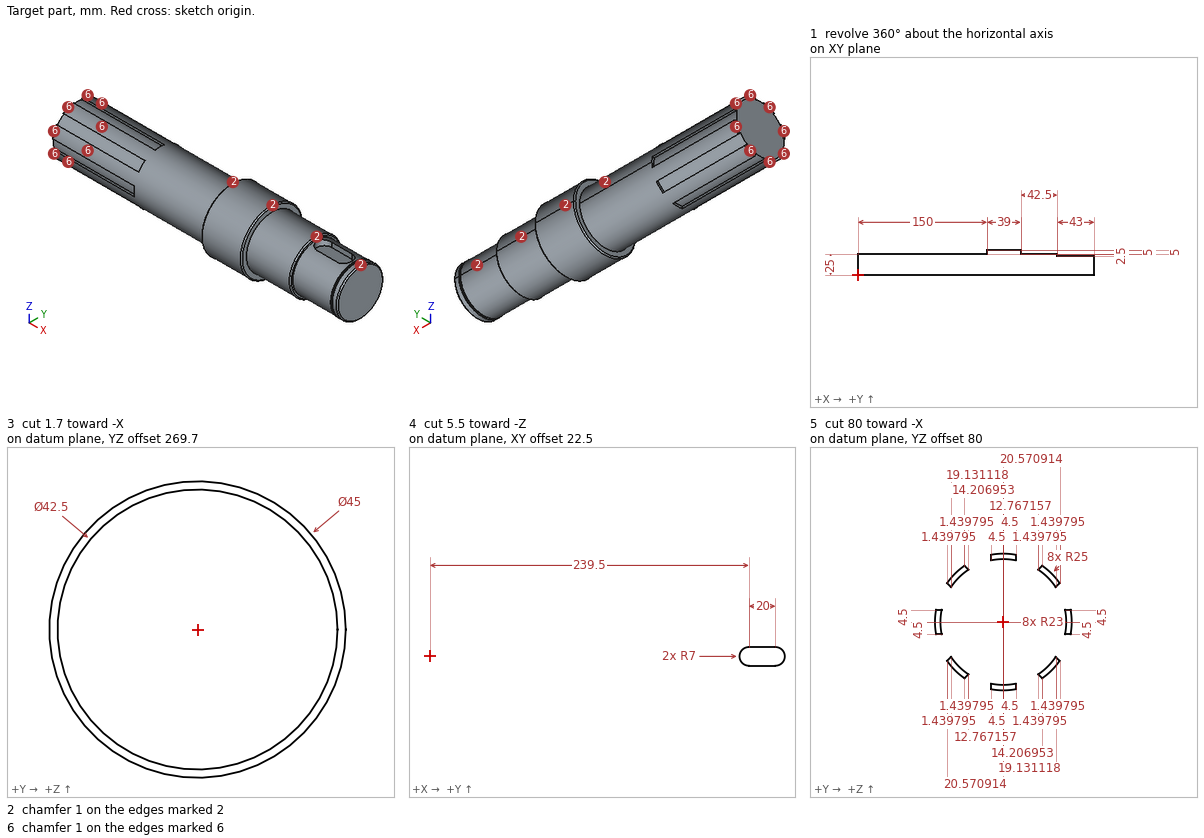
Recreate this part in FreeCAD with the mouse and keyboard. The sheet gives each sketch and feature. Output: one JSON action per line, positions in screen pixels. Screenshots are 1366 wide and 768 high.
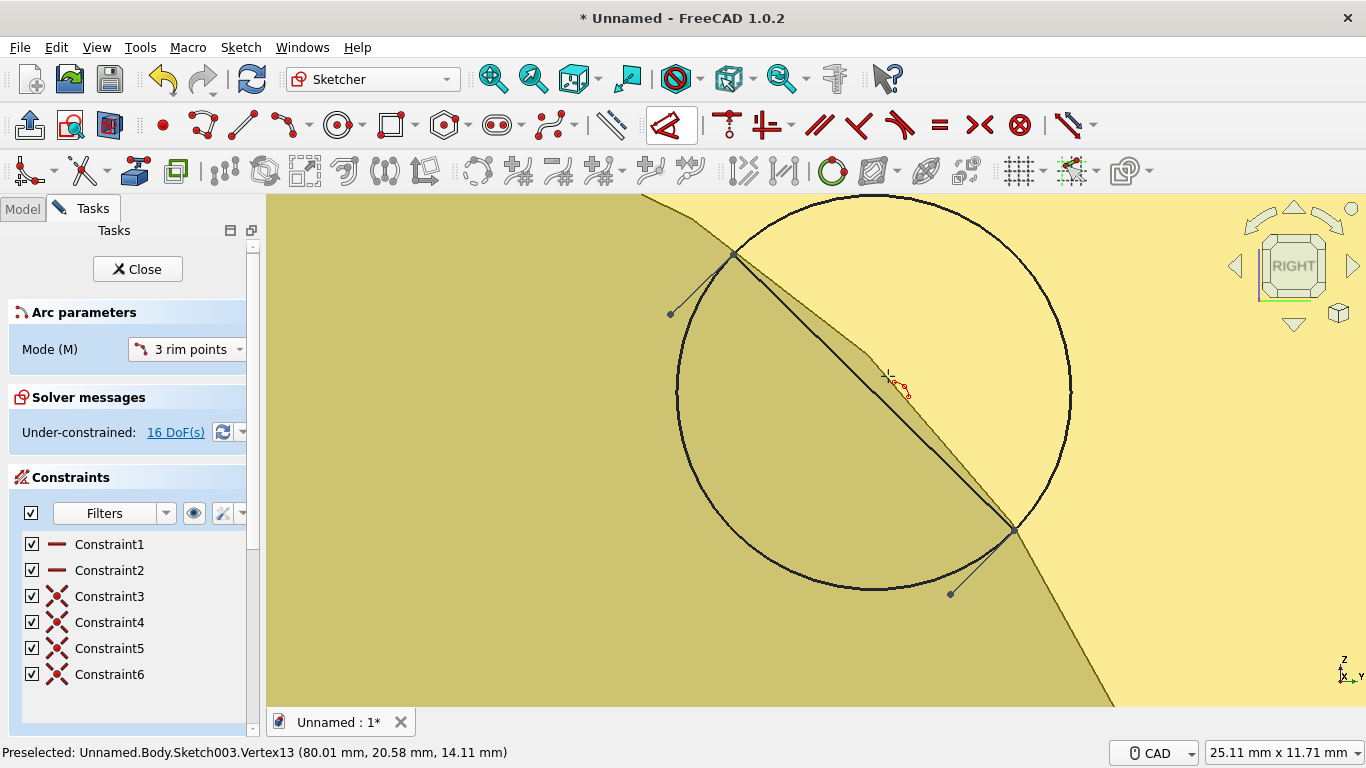
{"action": "left_click", "coordinate": [887, 374]}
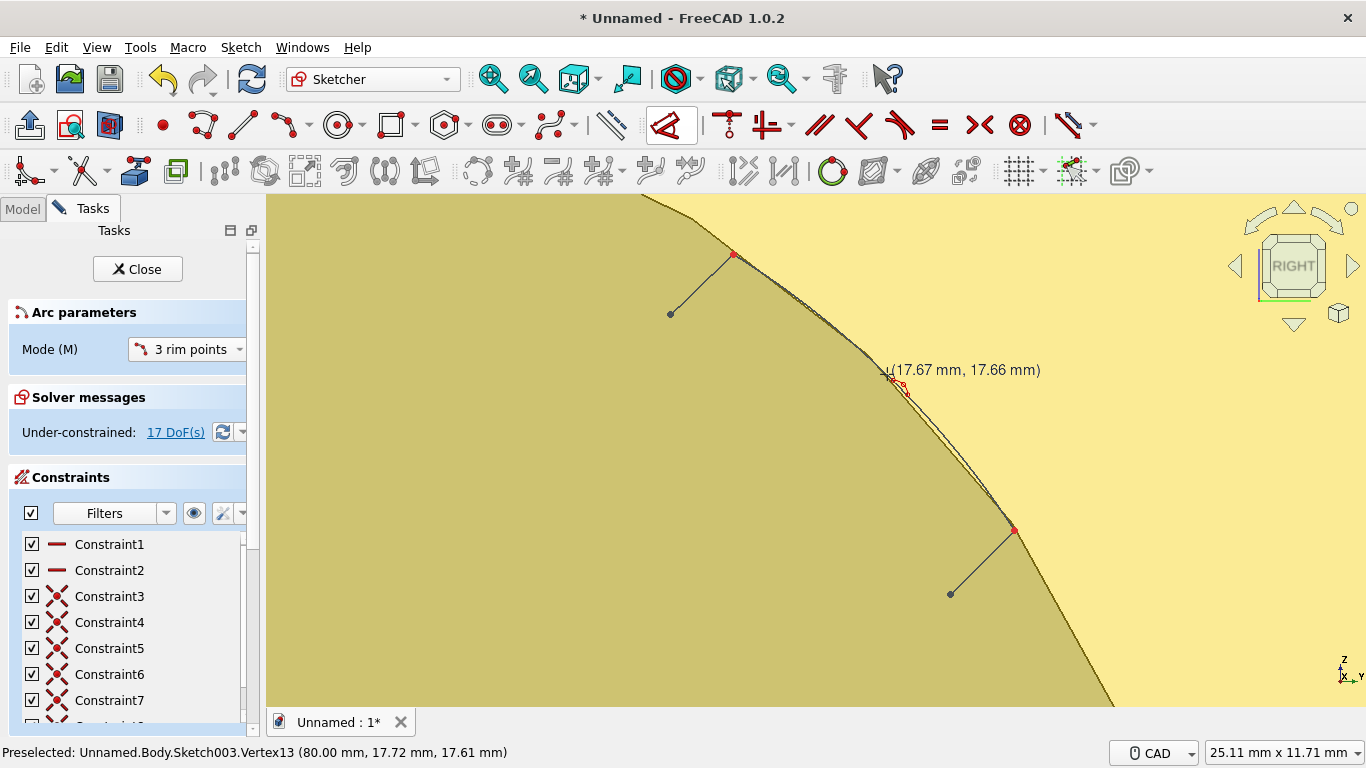
{"action": "left_click", "coordinate": [950, 595]}
{"action": "left_click", "coordinate": [671, 315]}
{"action": "left_click", "coordinate": [825, 436]}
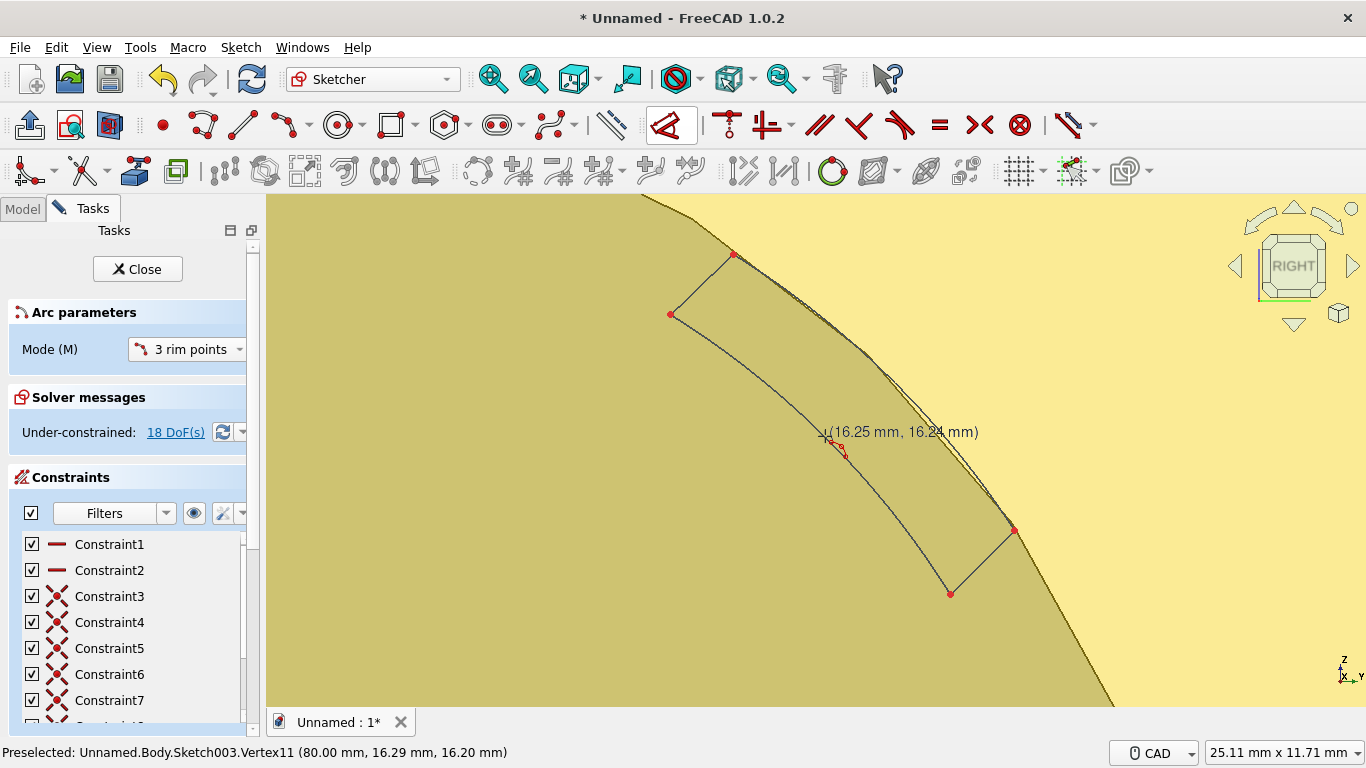
{"action": "left_click", "coordinate": [244, 126]}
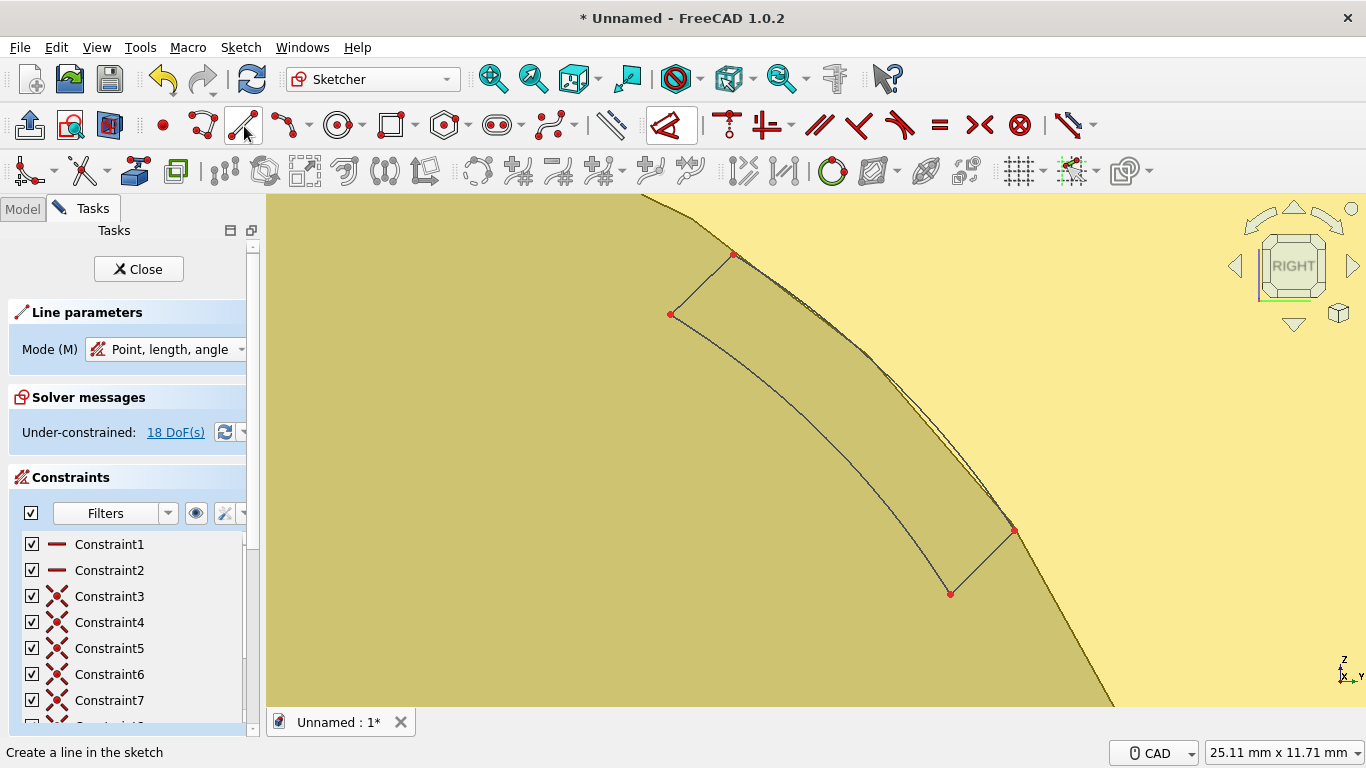
{"action": "scroll", "coordinate": [847, 341], "scroll_direction": "down", "scroll_amount": 10}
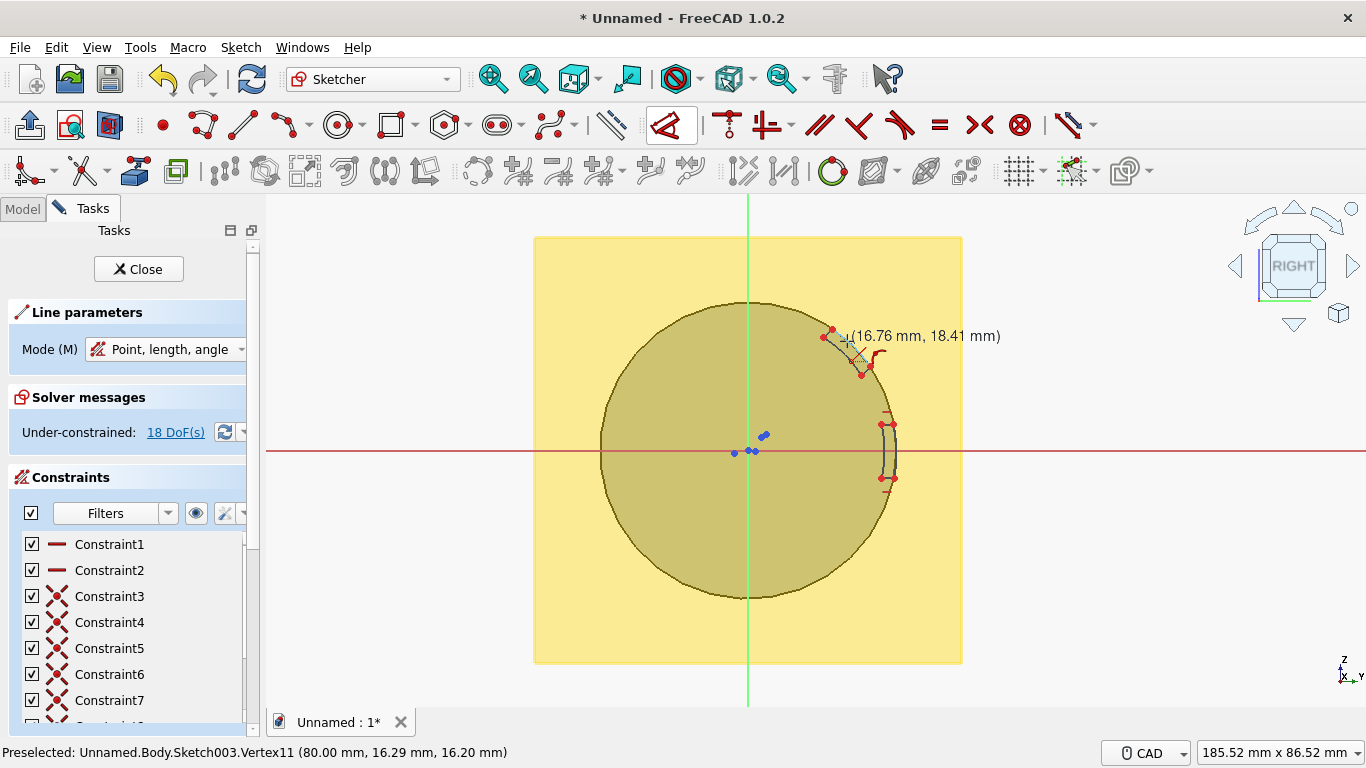
{"action": "left_click", "coordinate": [721, 317]}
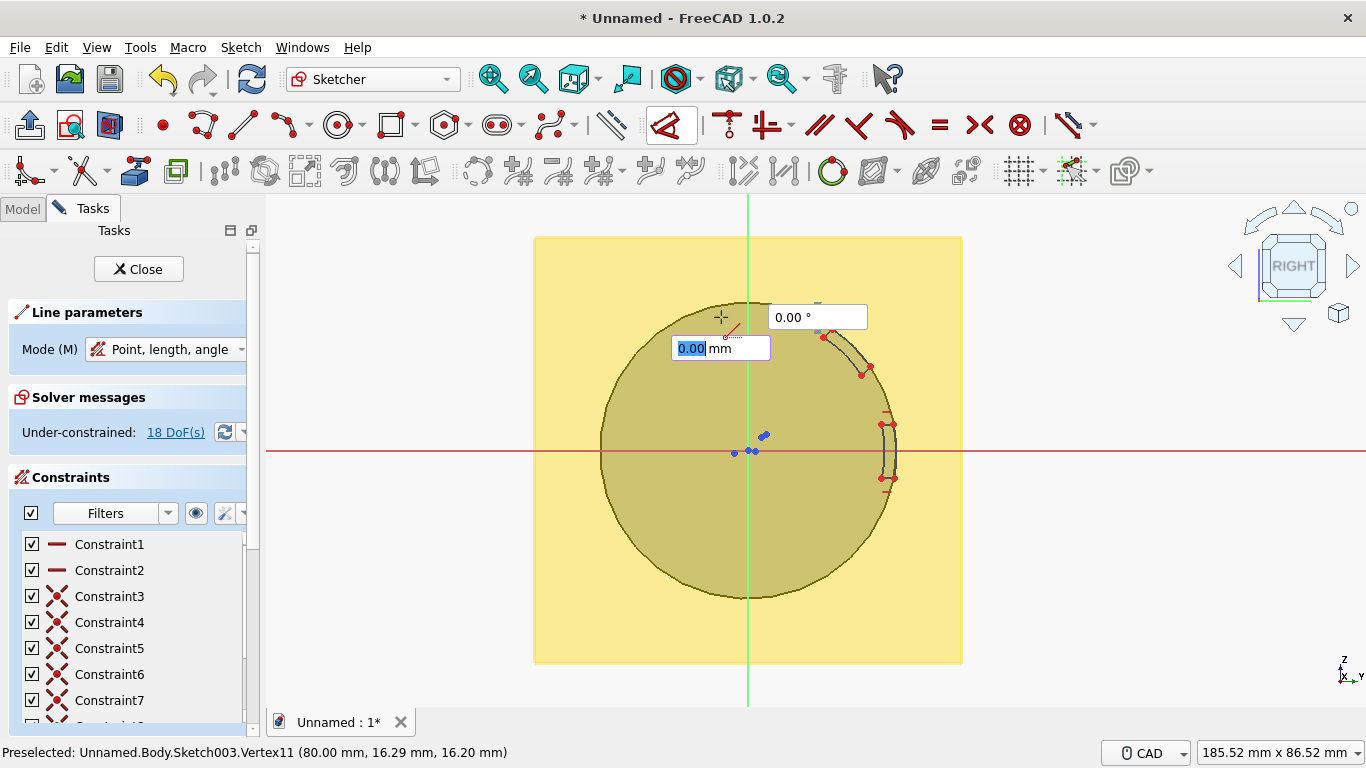
{"action": "scroll", "coordinate": [721, 305], "scroll_direction": "up", "scroll_amount": 2}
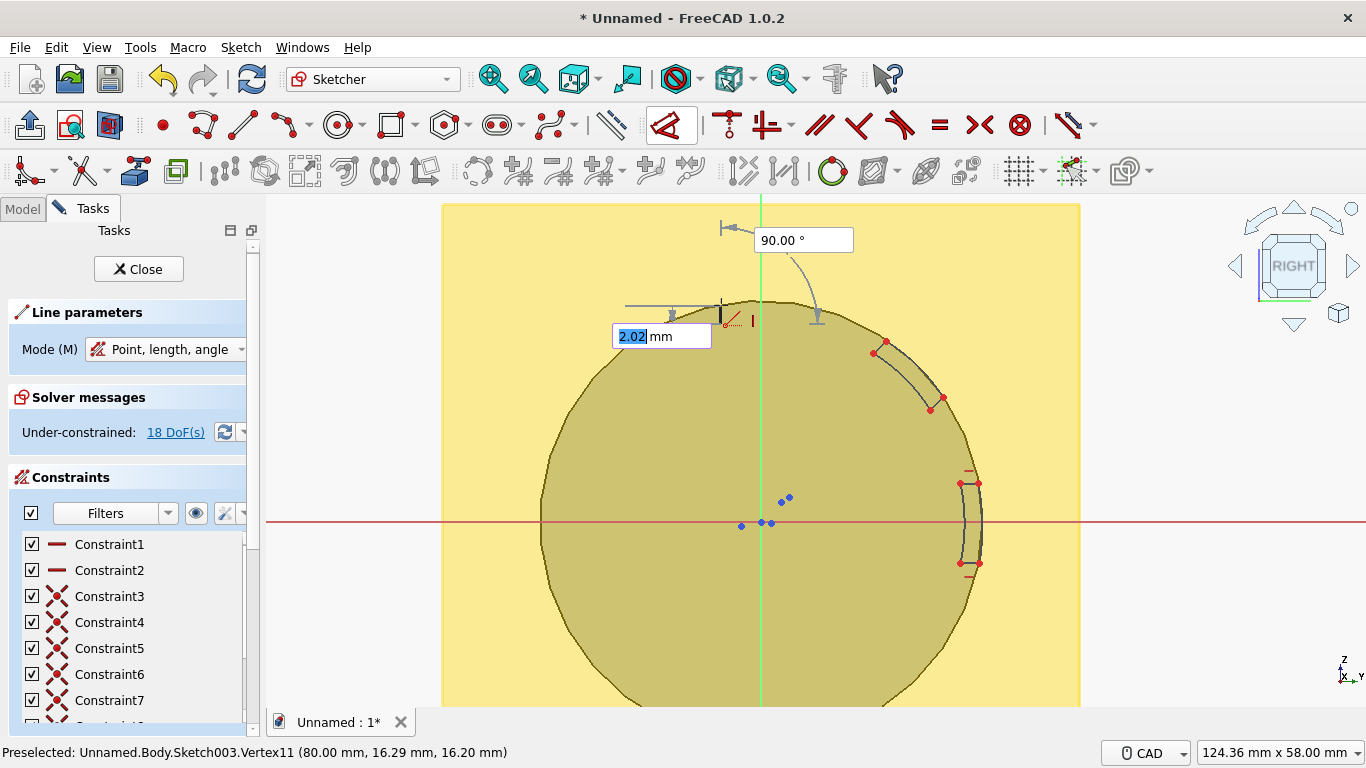
{"action": "left_click", "coordinate": [721, 305]}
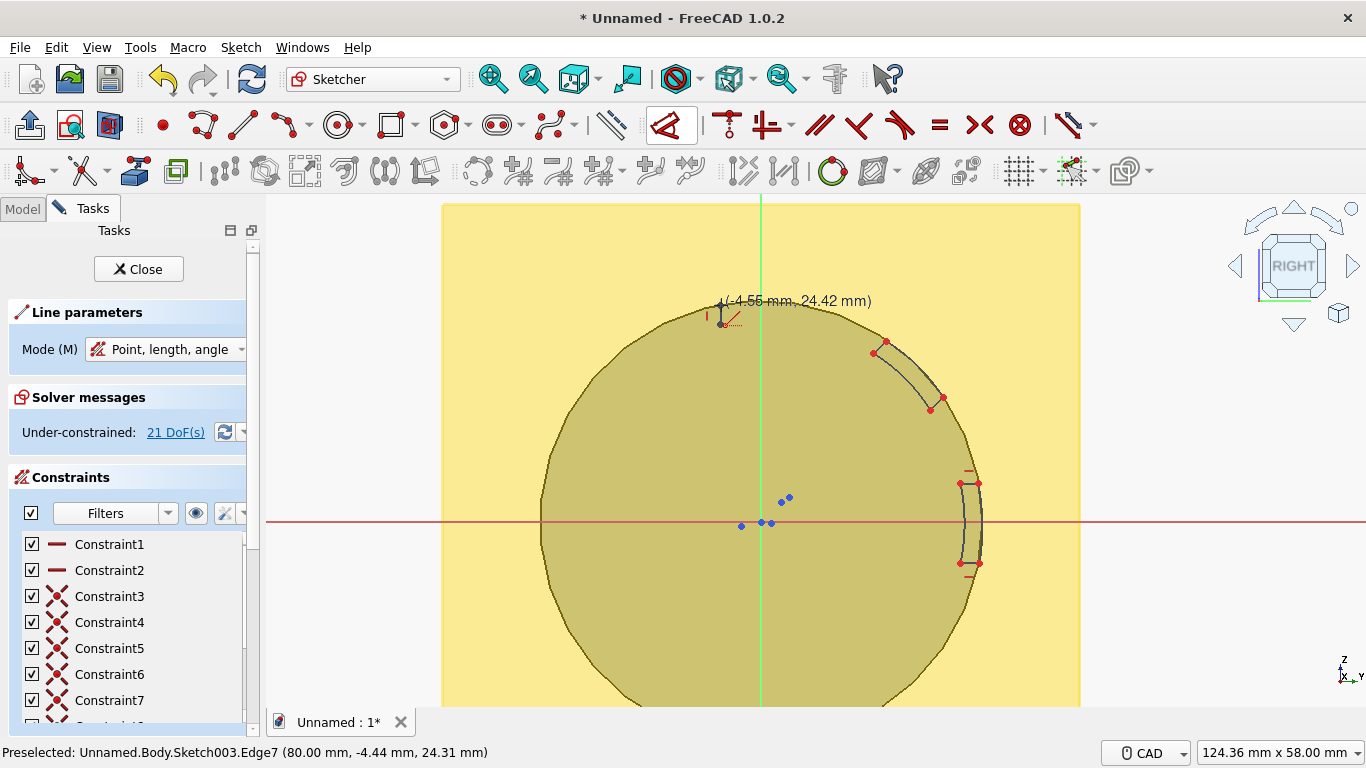
{"action": "left_click", "coordinate": [801, 305]}
{"action": "left_click", "coordinate": [801, 323]}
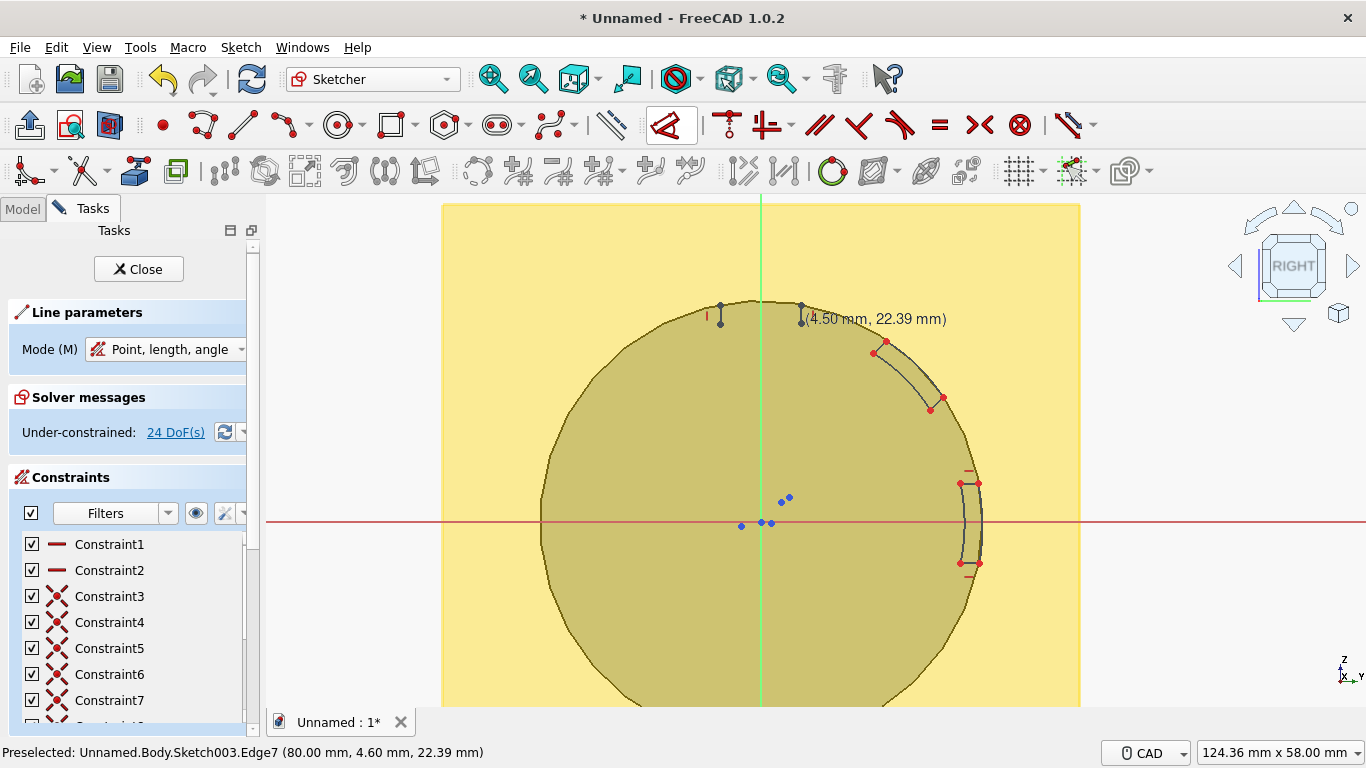
{"action": "left_click", "coordinate": [284, 126]}